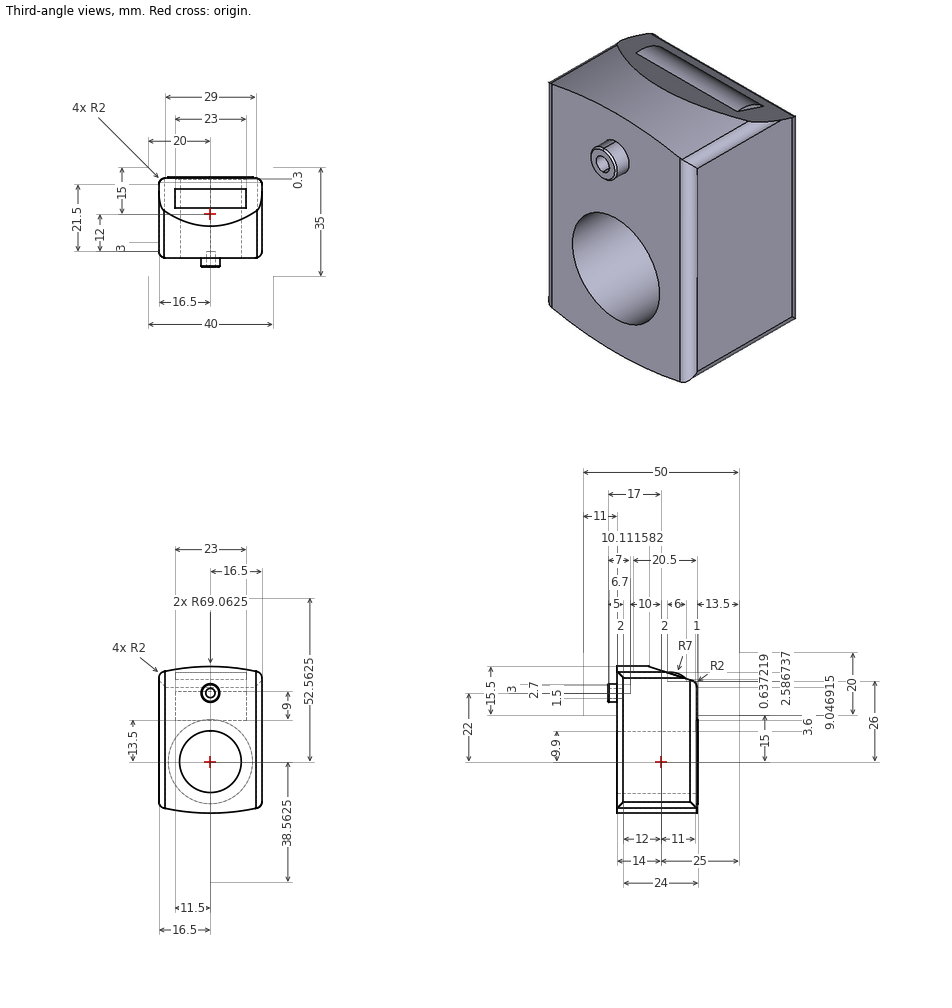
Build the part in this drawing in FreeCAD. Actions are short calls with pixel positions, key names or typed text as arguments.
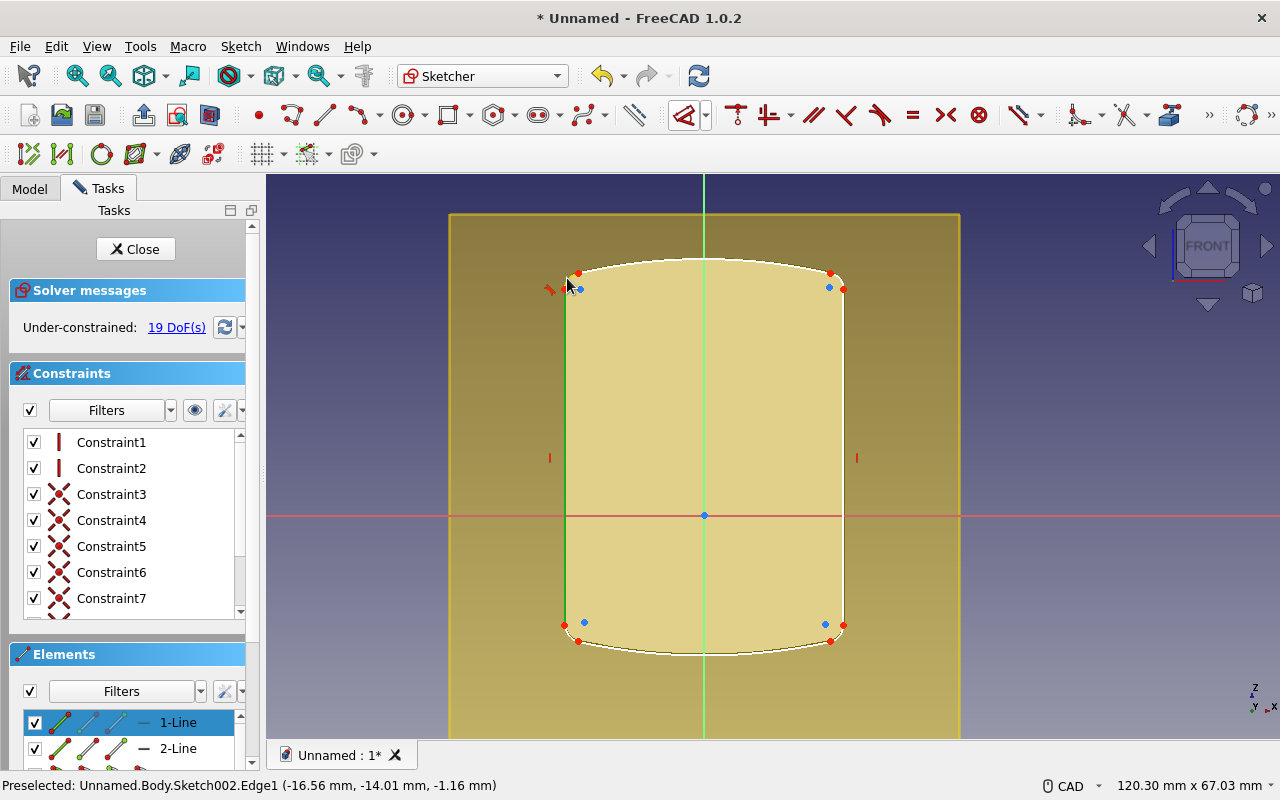
scroll(567, 632, up, 4)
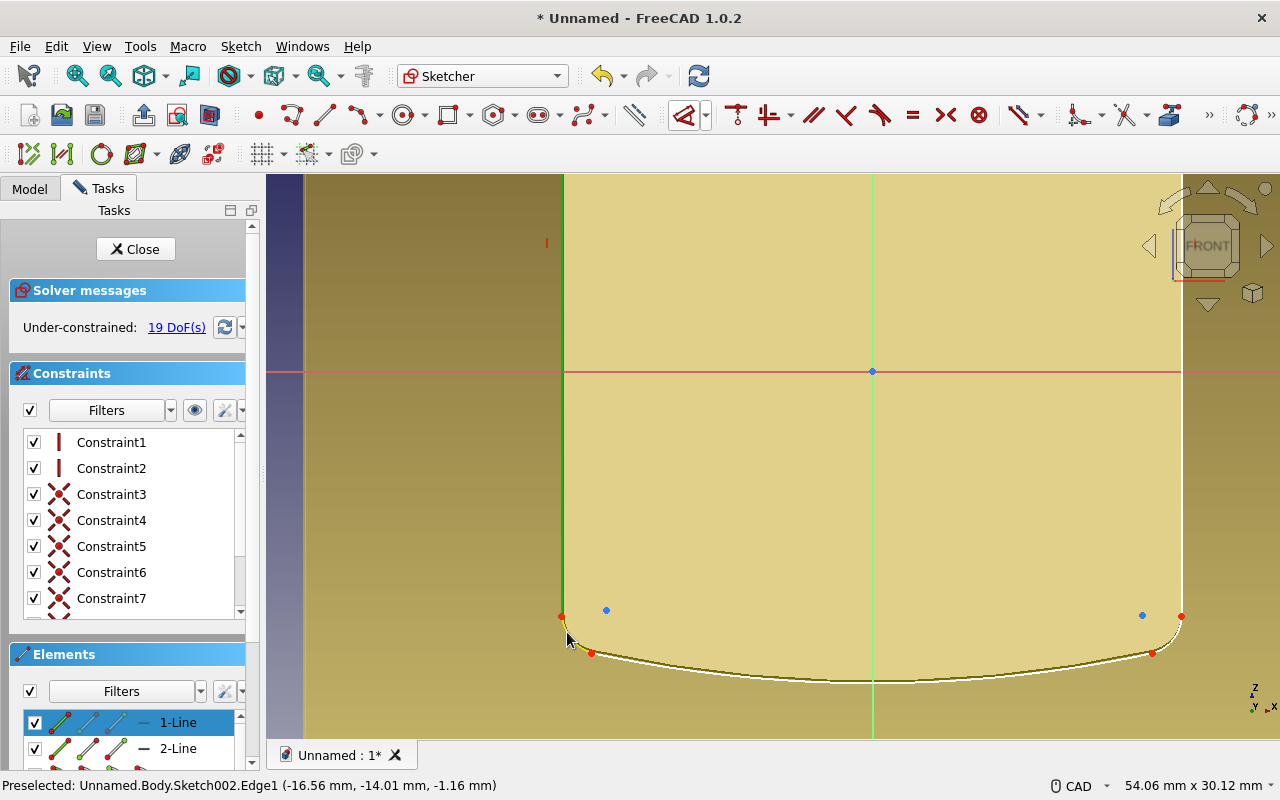
click(566, 631)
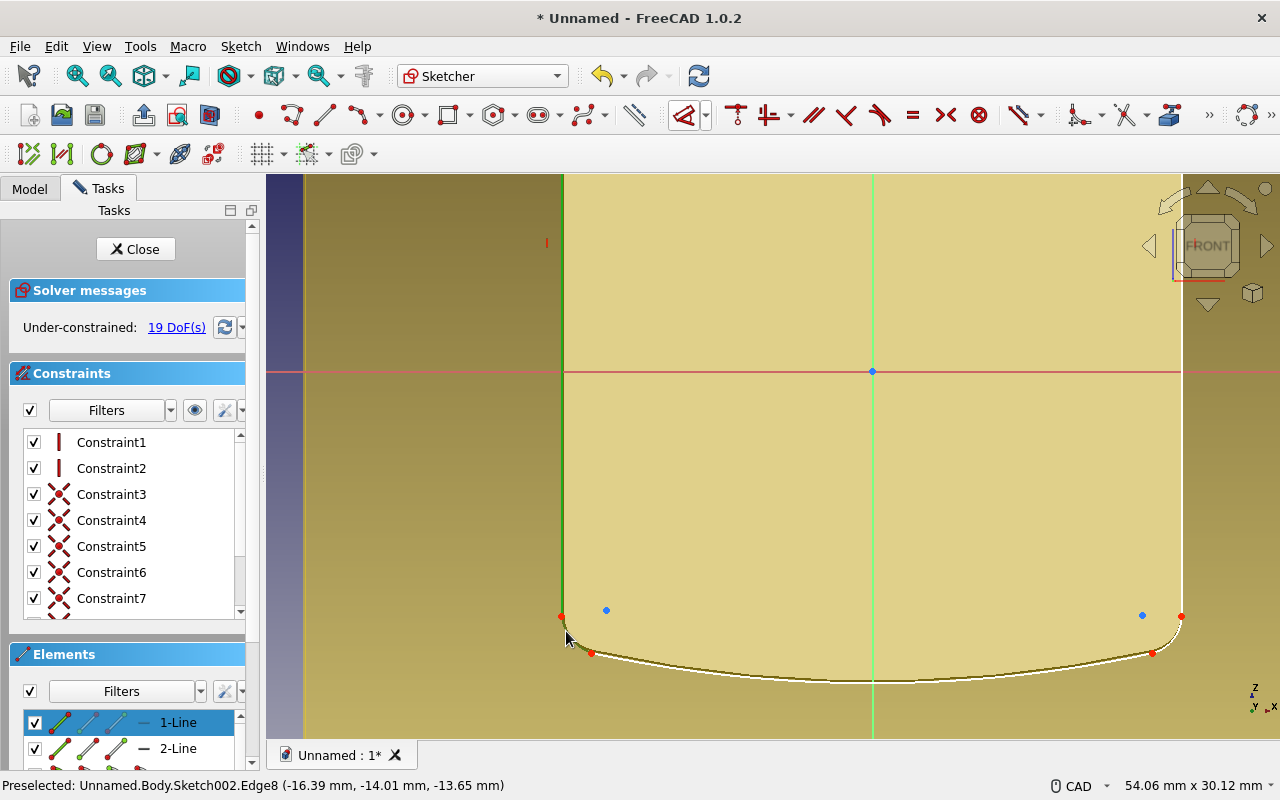
click(880, 116)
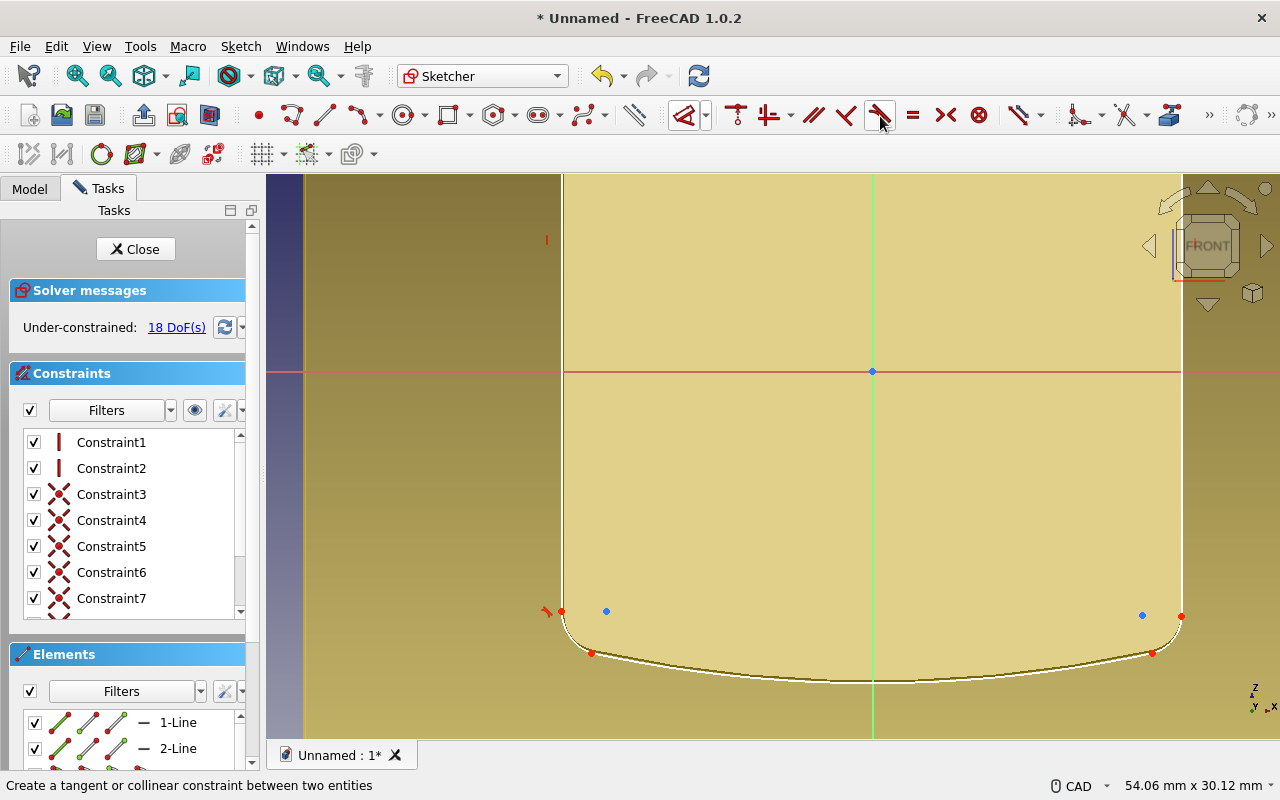
scroll(567, 633, down, 4)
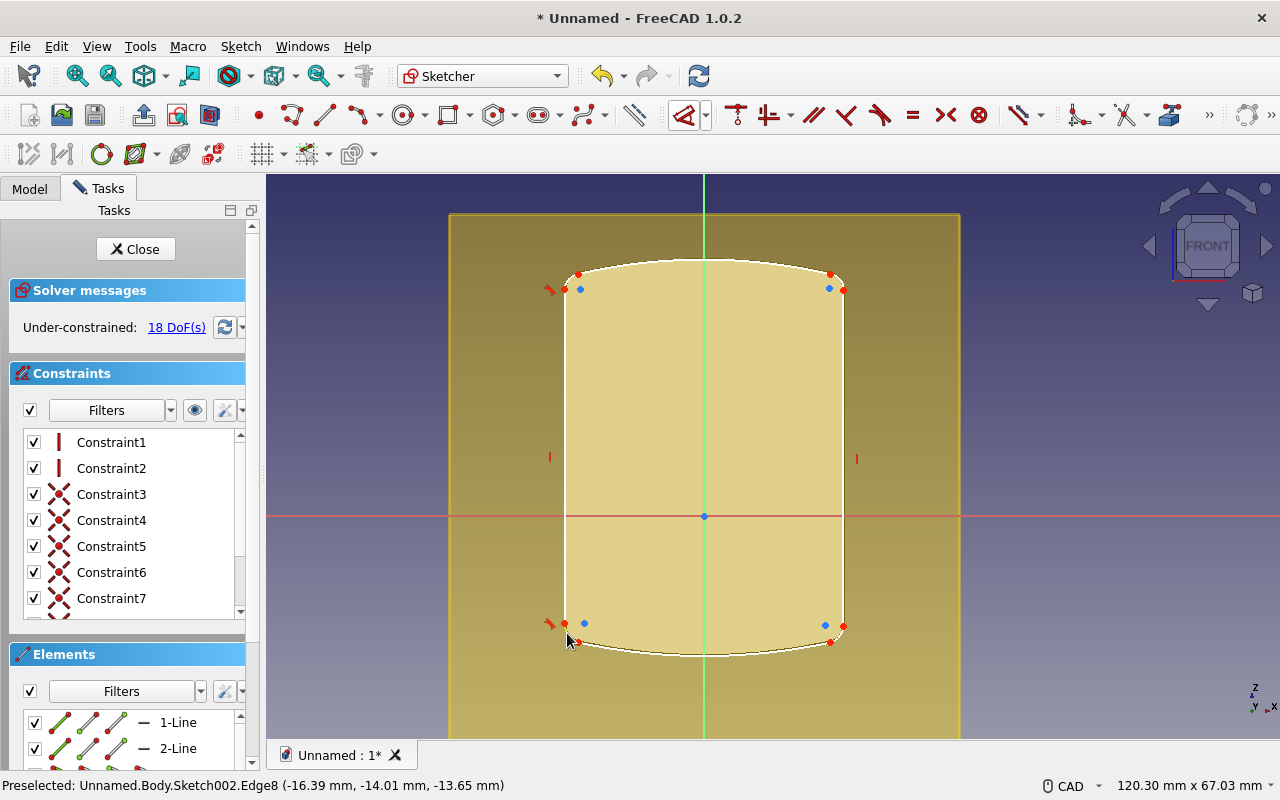
click(843, 391)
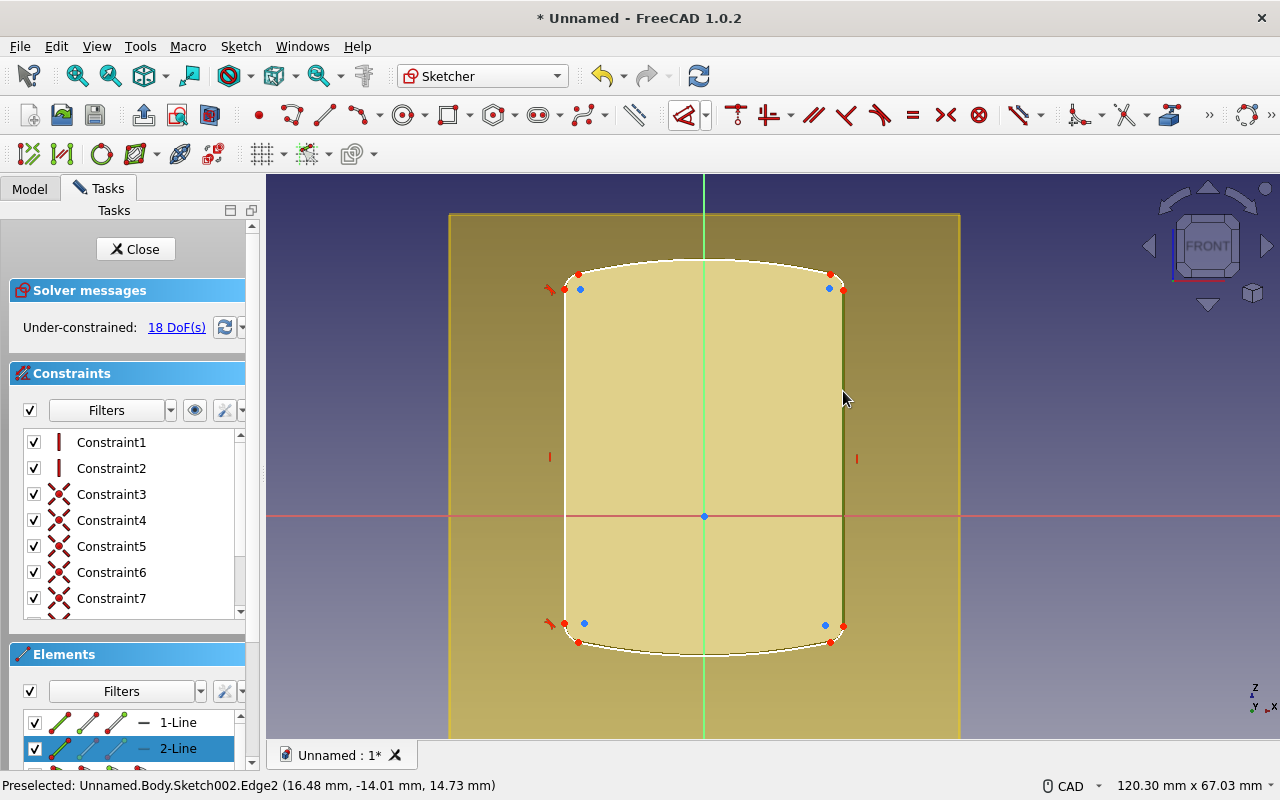
scroll(840, 279, up, 2)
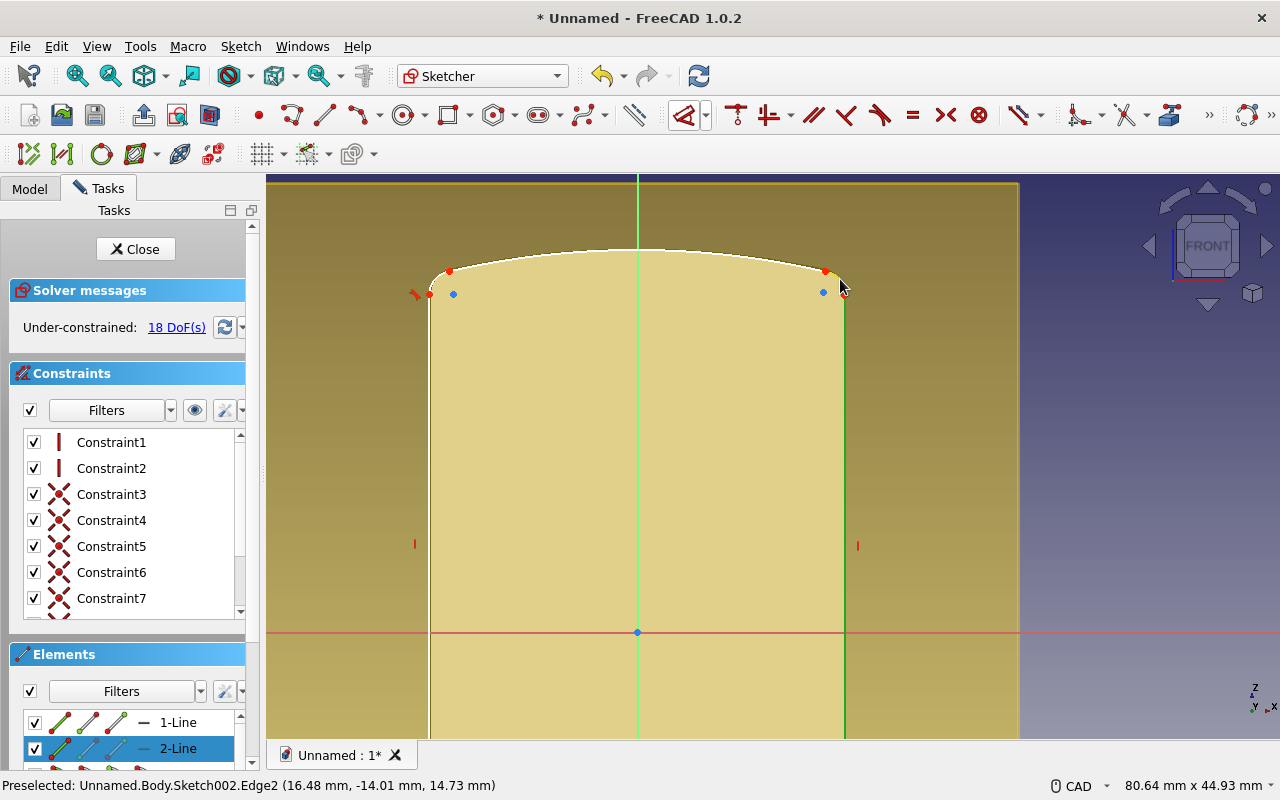
click(840, 279)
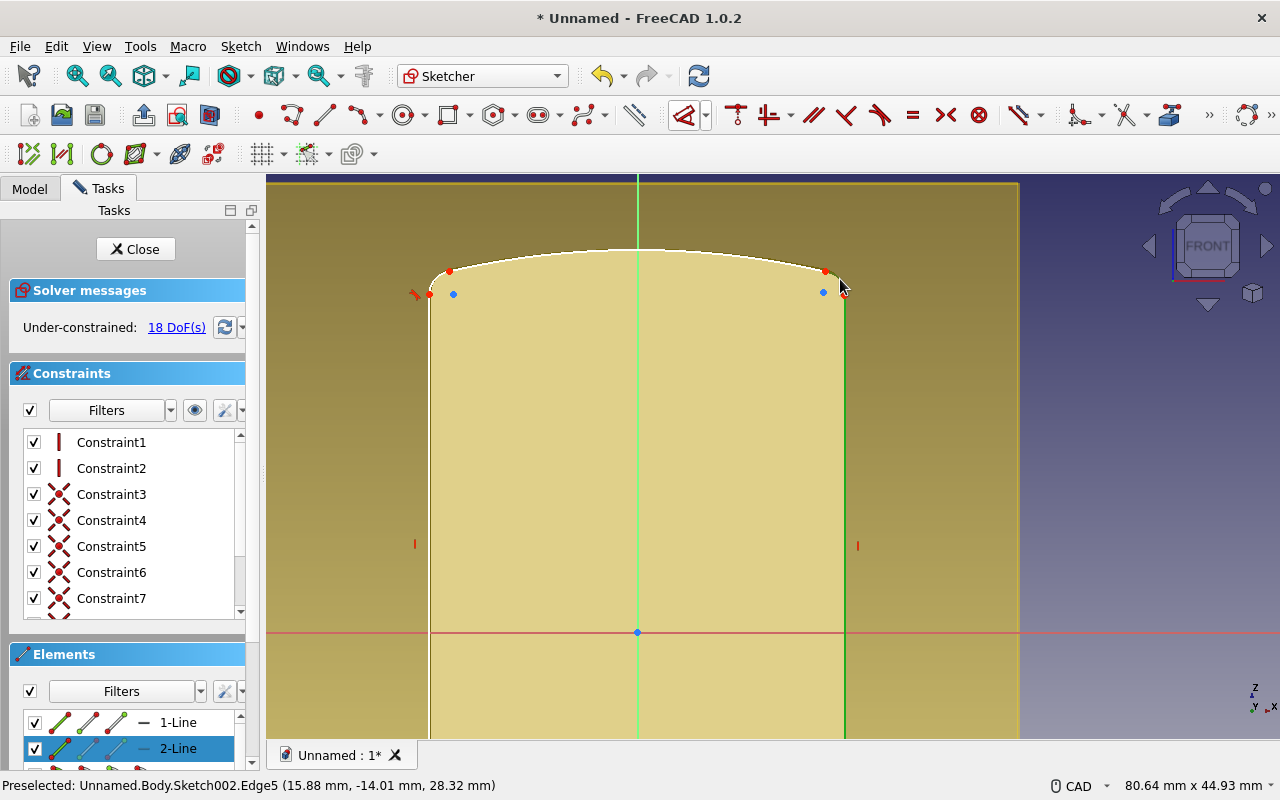
click(880, 116)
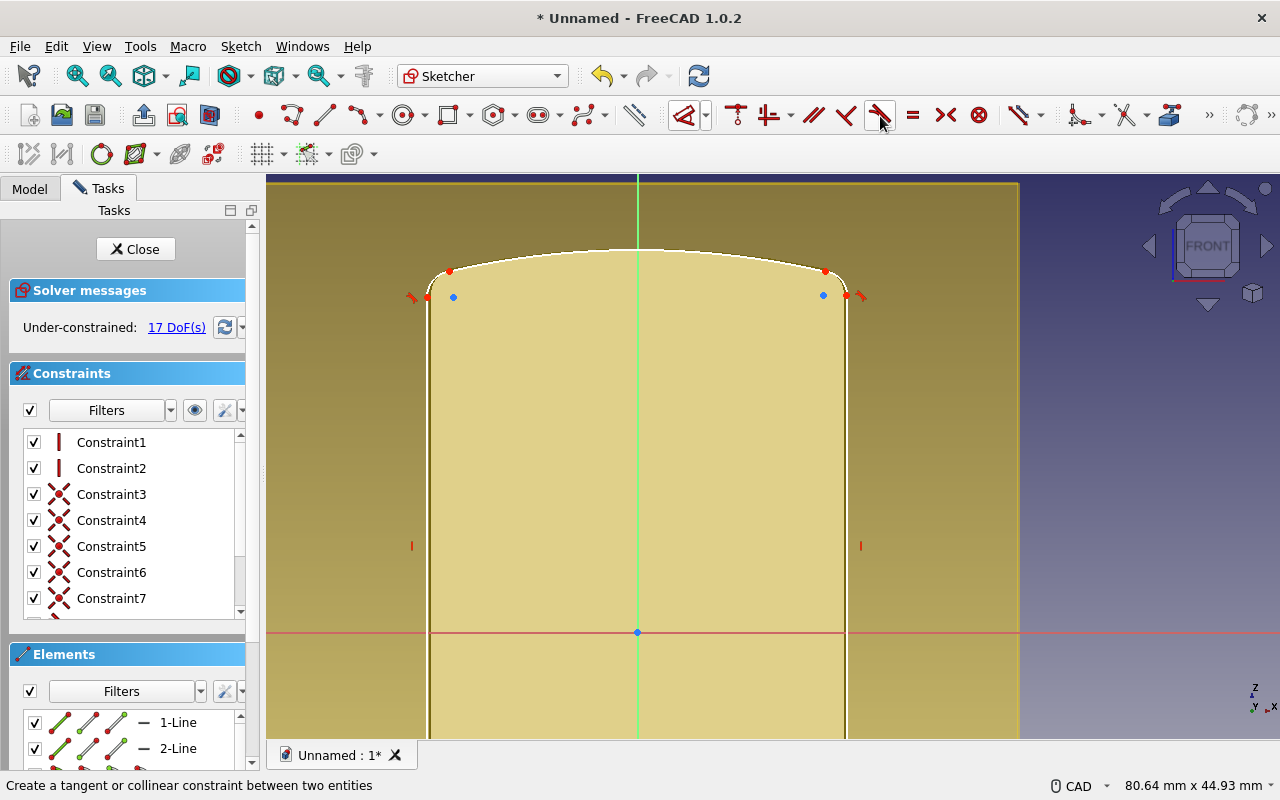
click(847, 446)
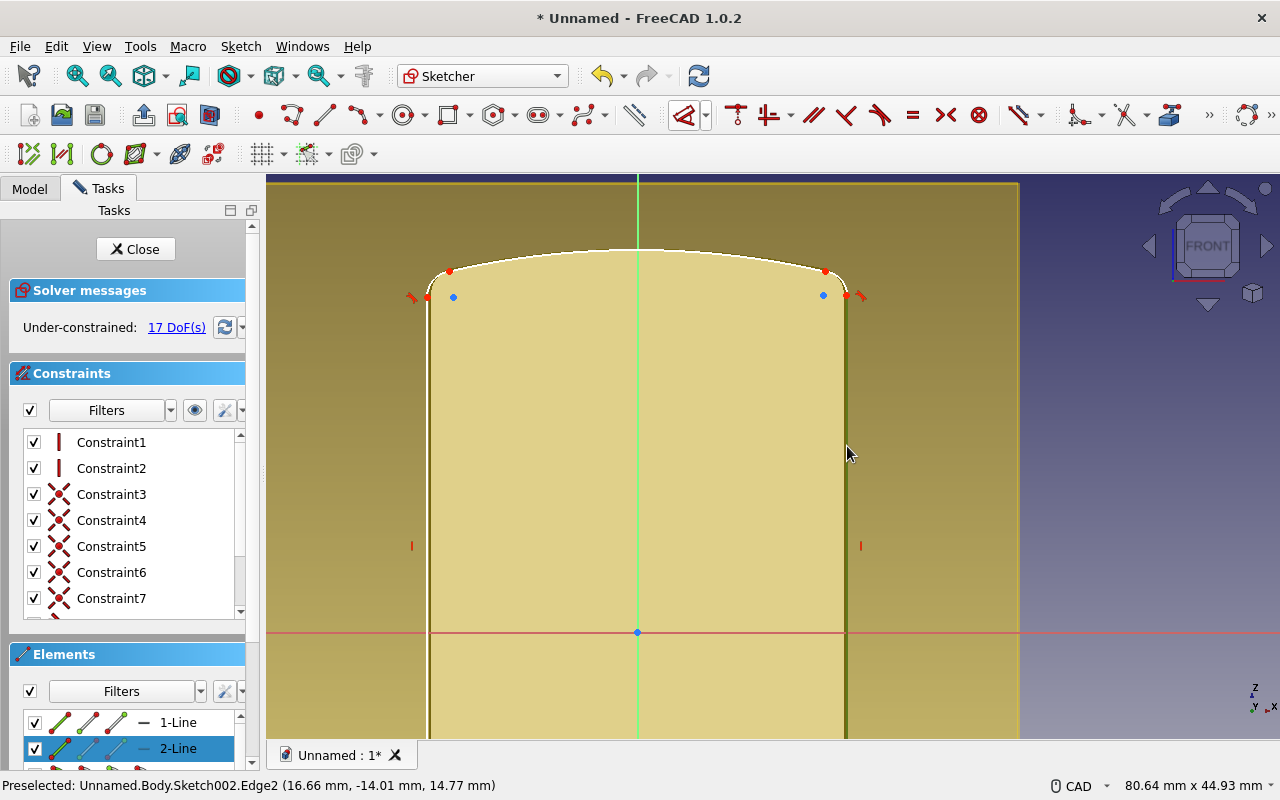
scroll(841, 277, down, 2)